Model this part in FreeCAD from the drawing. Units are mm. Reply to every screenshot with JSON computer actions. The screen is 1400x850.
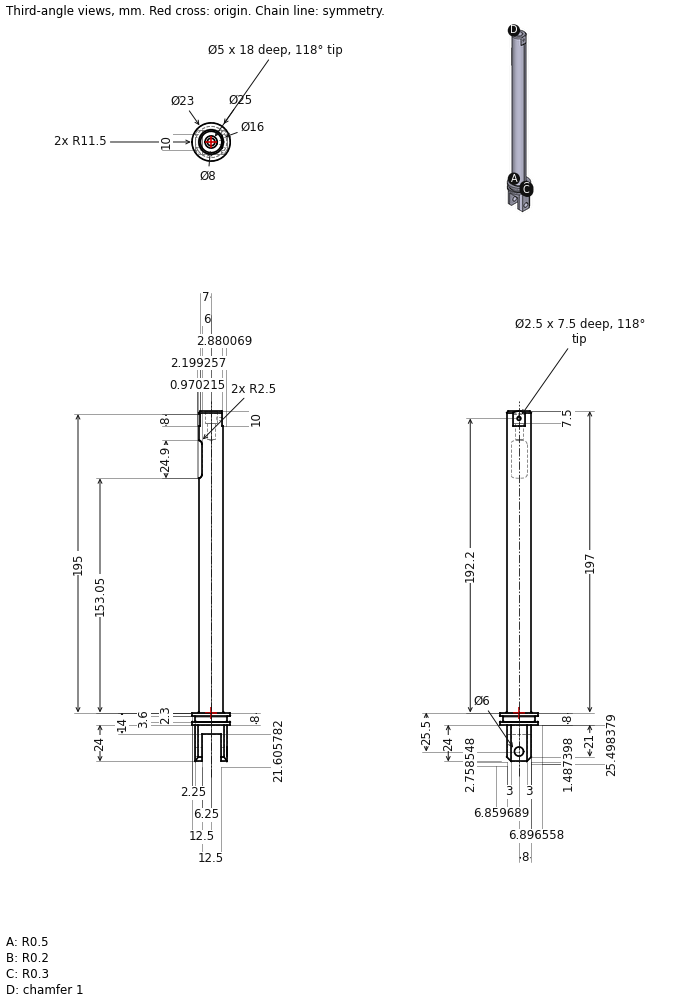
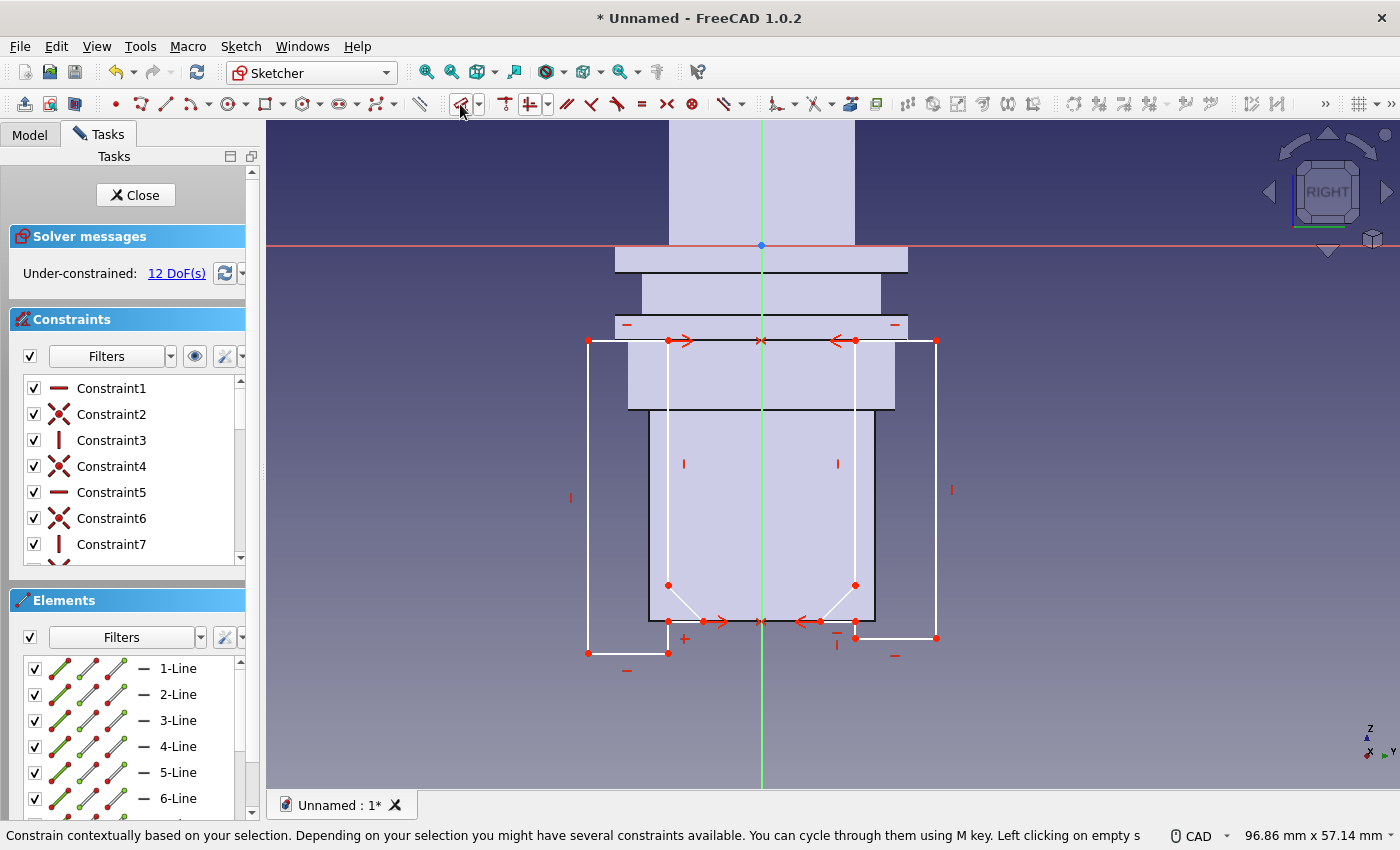
{"action": "scroll", "coordinate": [844, 622], "scroll_direction": "up", "scroll_amount": 2}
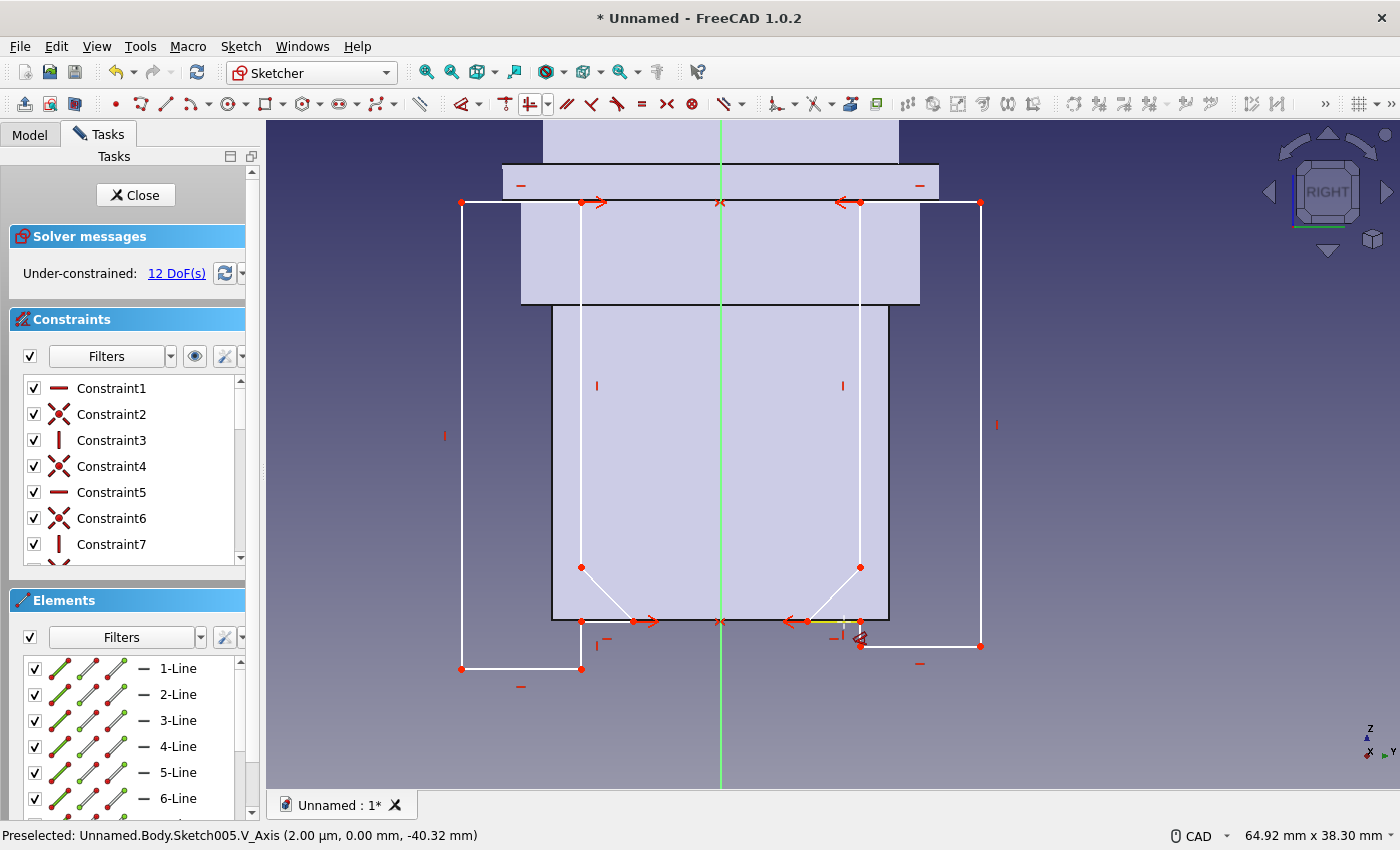
{"action": "left_click", "coordinate": [844, 622]}
{"action": "left_click", "coordinate": [834, 656]}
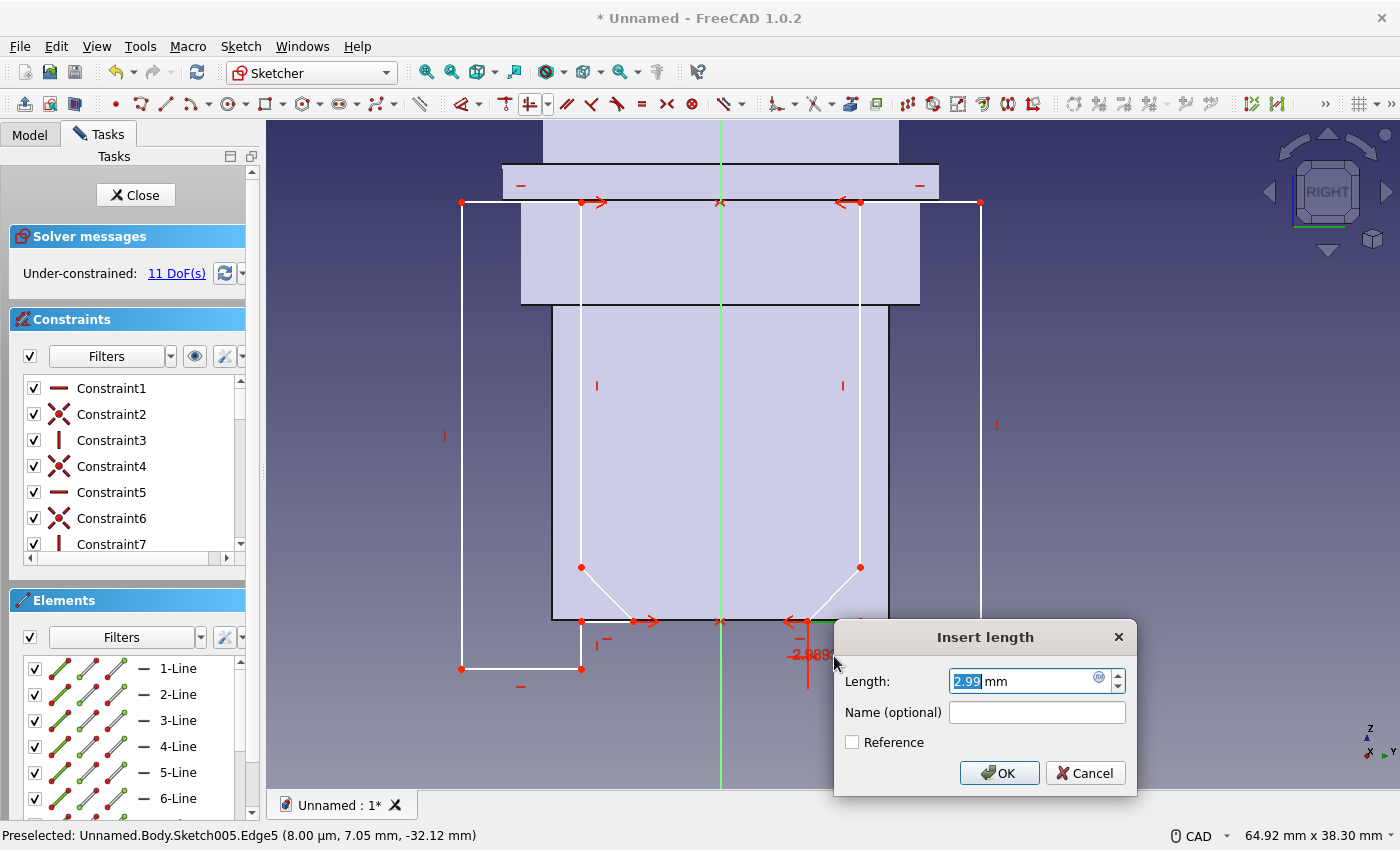
{"action": "type", "text": "3"}
{"action": "key", "text": "Return"}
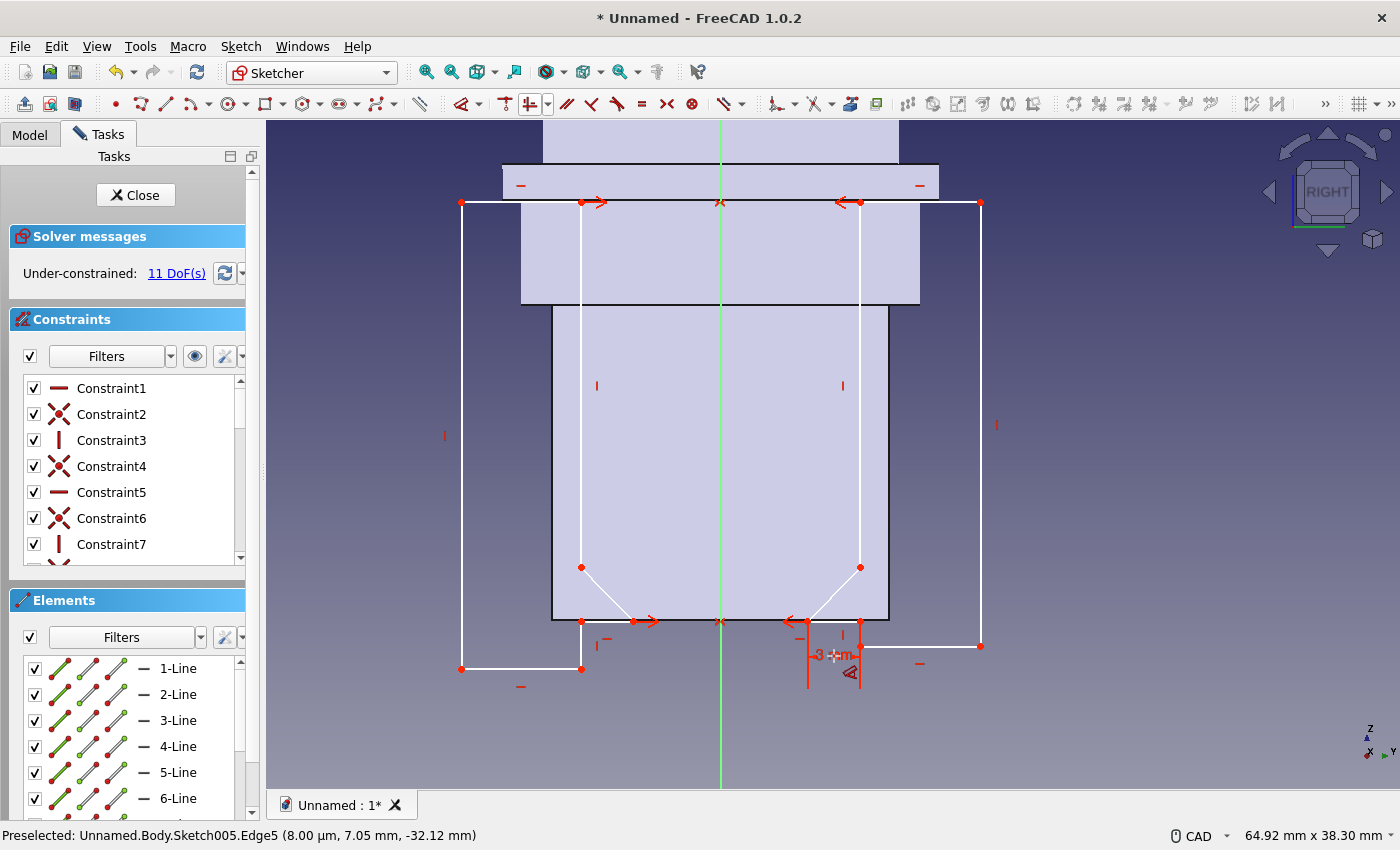
{"action": "scroll", "coordinate": [618, 622], "scroll_direction": "up", "scroll_amount": 2}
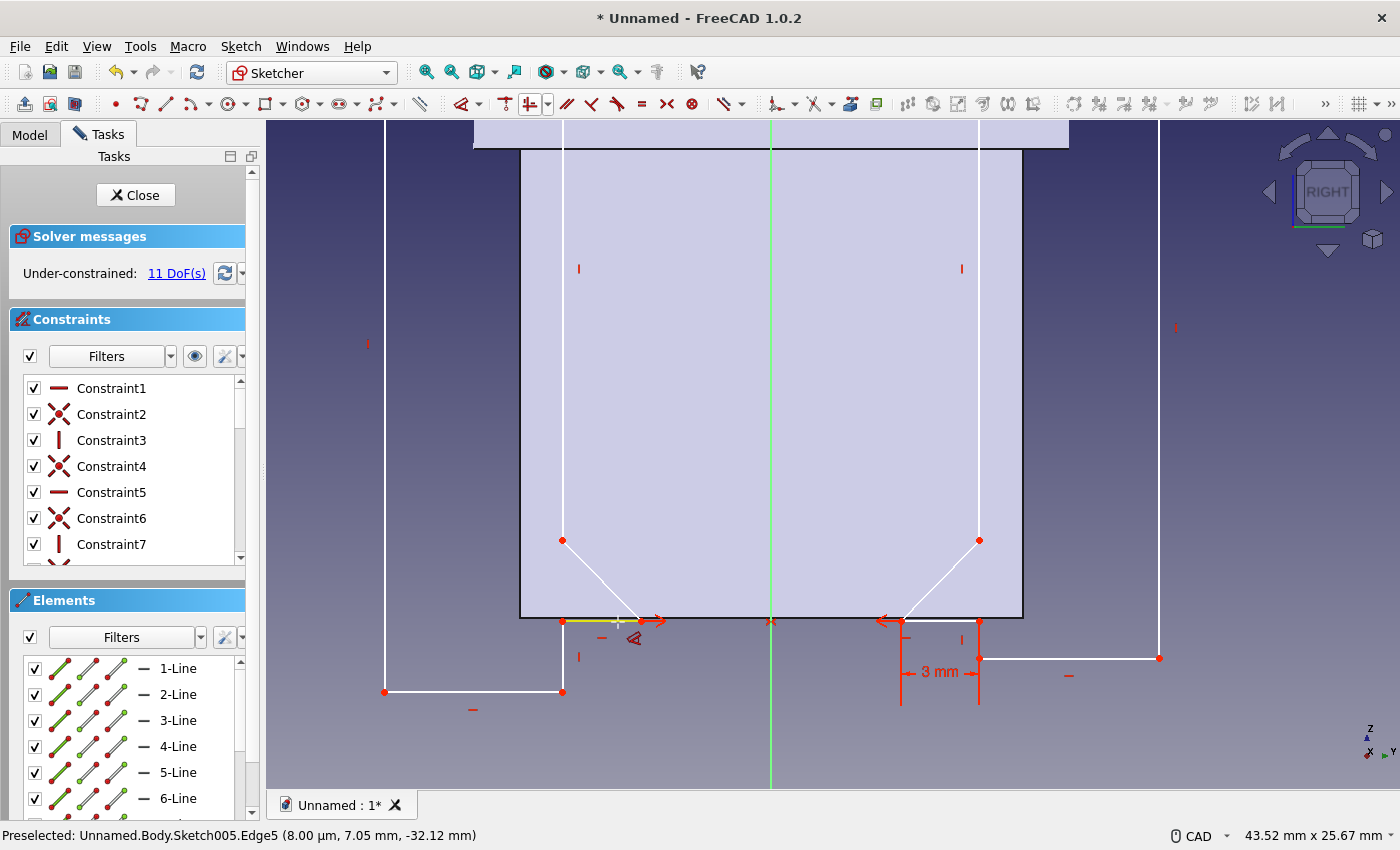
{"action": "left_click", "coordinate": [618, 621]}
{"action": "left_click", "coordinate": [602, 655]}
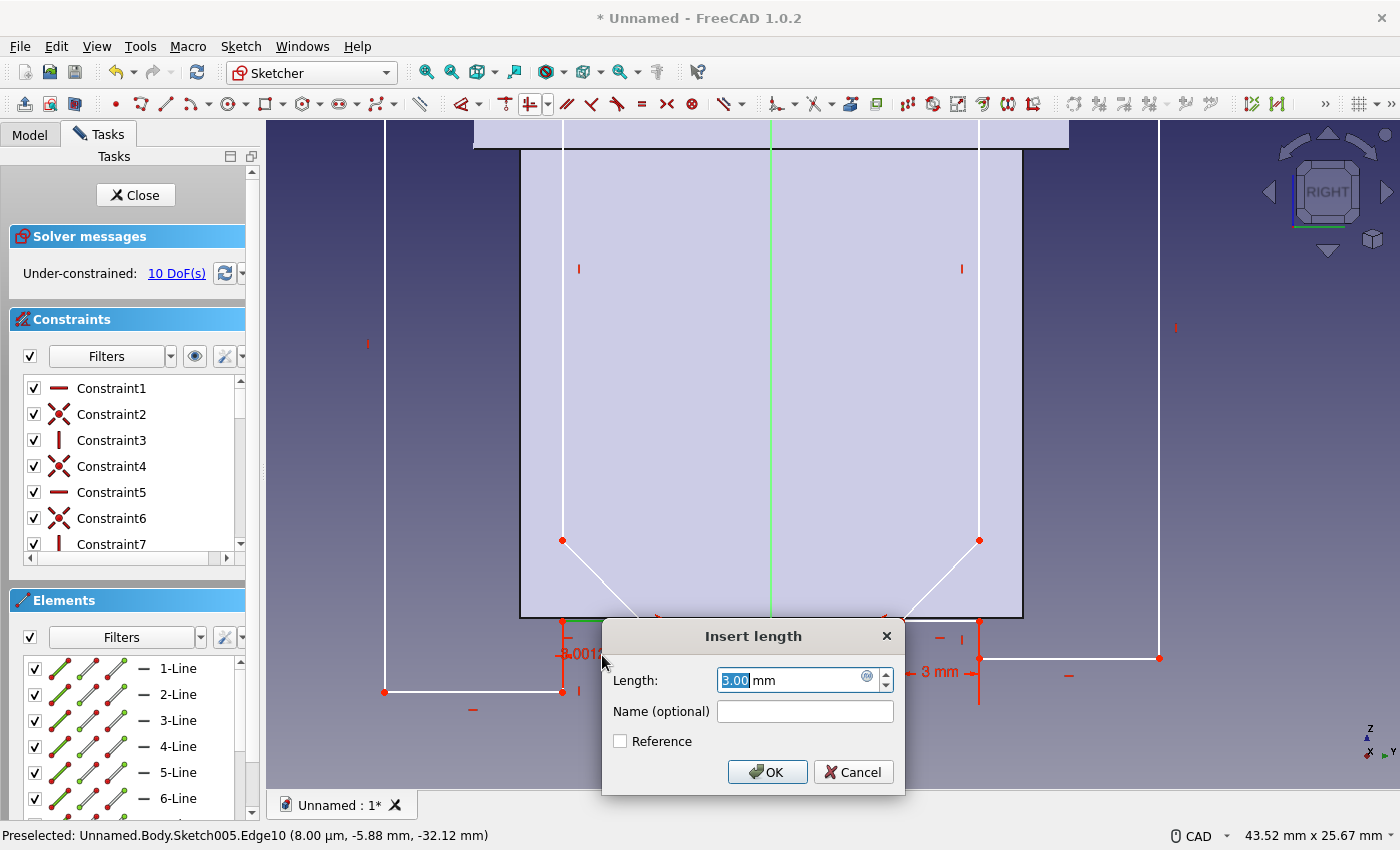
{"action": "type", "text": "3"}
{"action": "key", "text": "Return"}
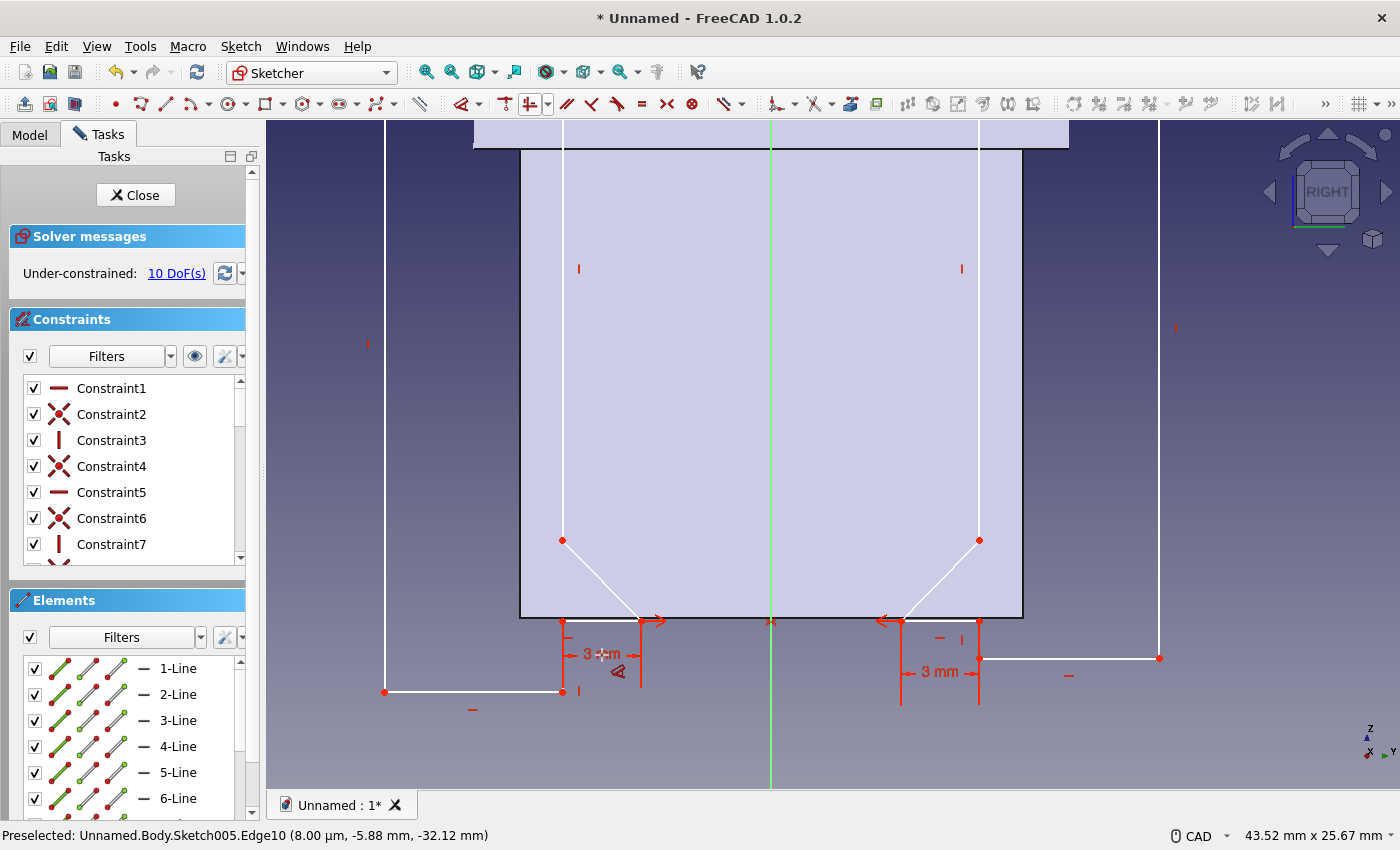
{"action": "left_click", "coordinate": [979, 377]}
{"action": "left_click", "coordinate": [1013, 344]}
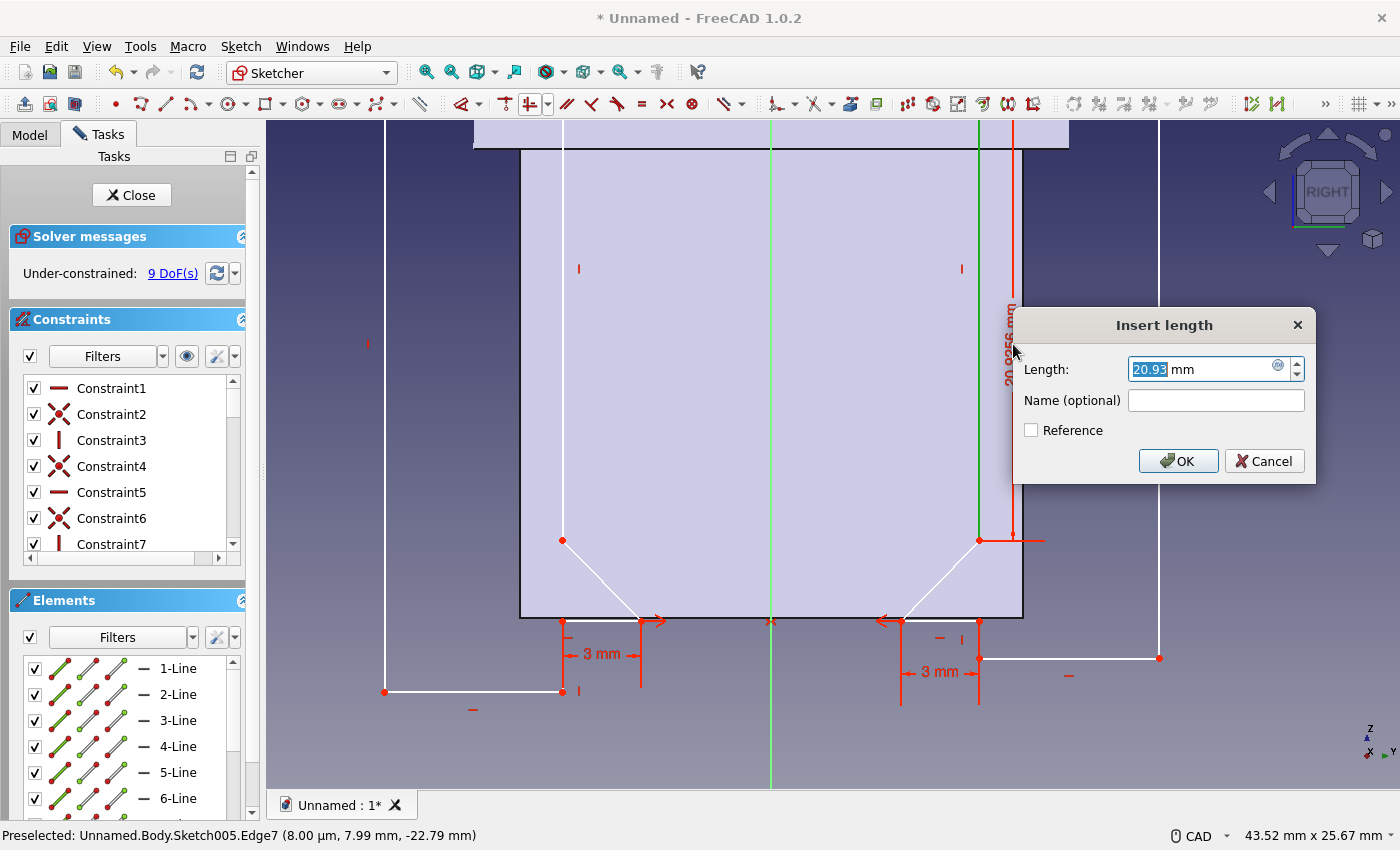
{"action": "type", "text": "21"}
{"action": "key", "text": "Return"}